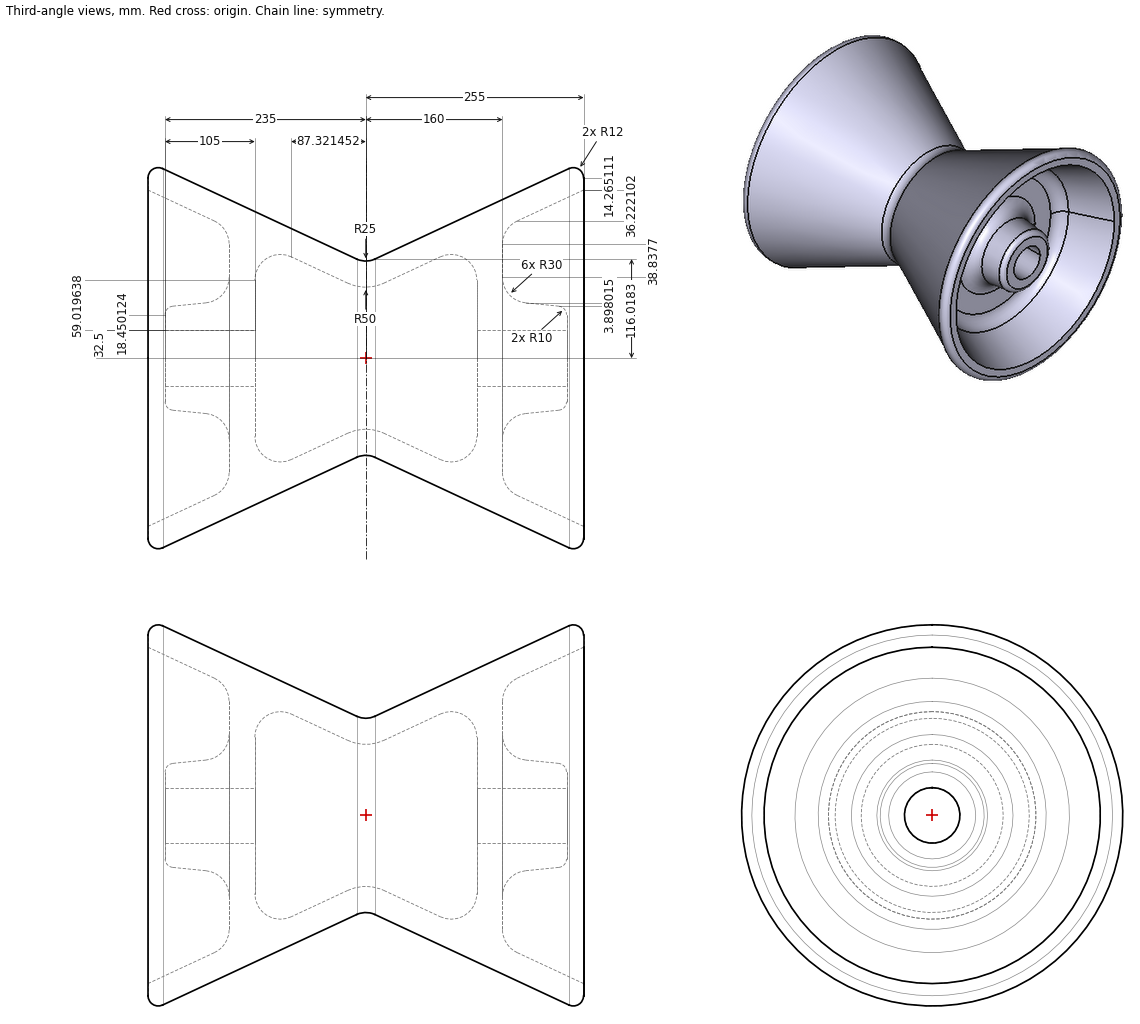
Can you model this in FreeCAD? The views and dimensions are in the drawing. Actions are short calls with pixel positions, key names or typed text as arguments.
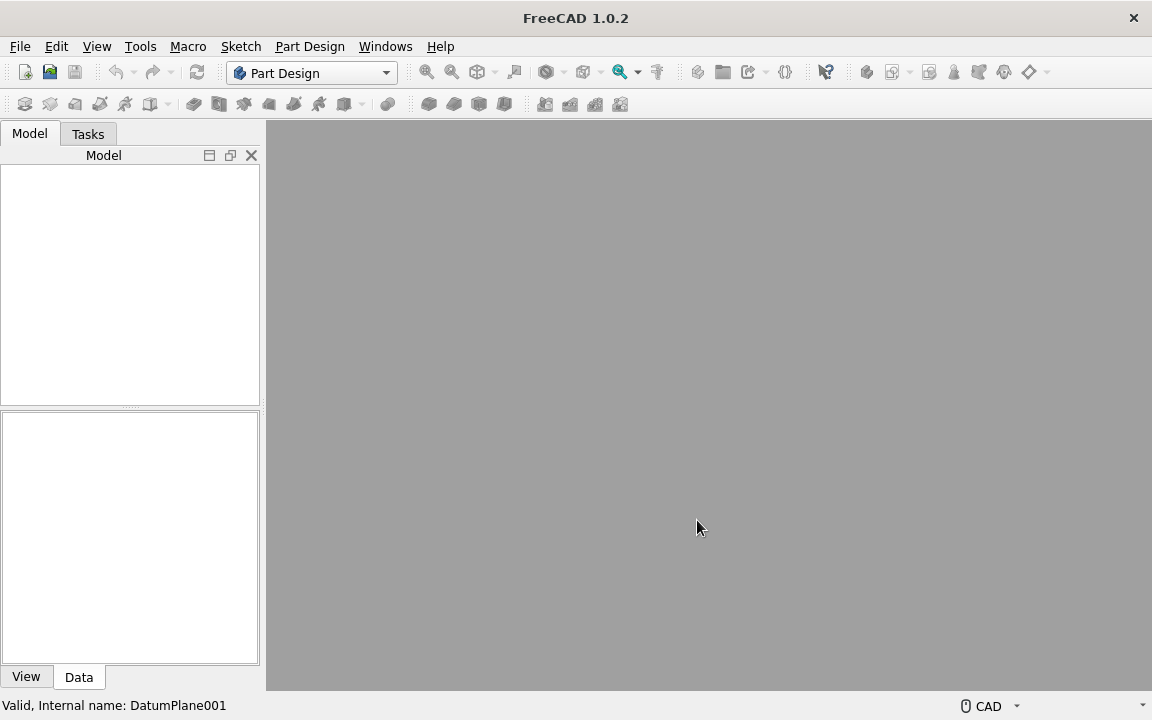
click(25, 72)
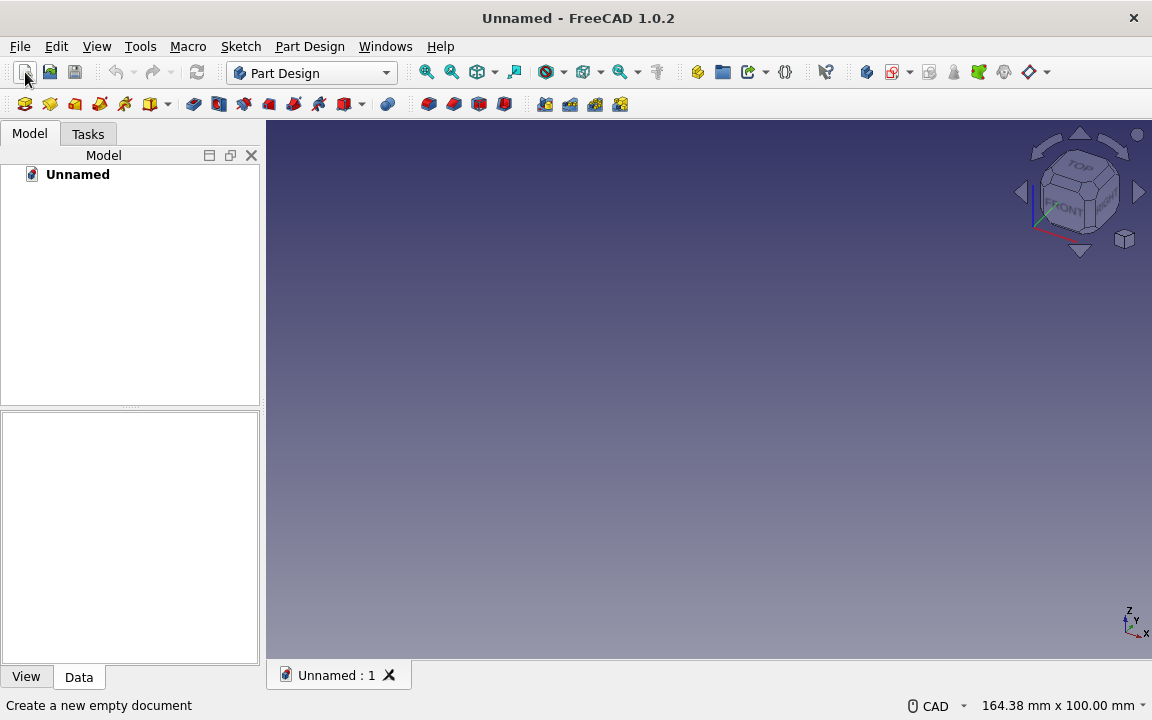
click(892, 72)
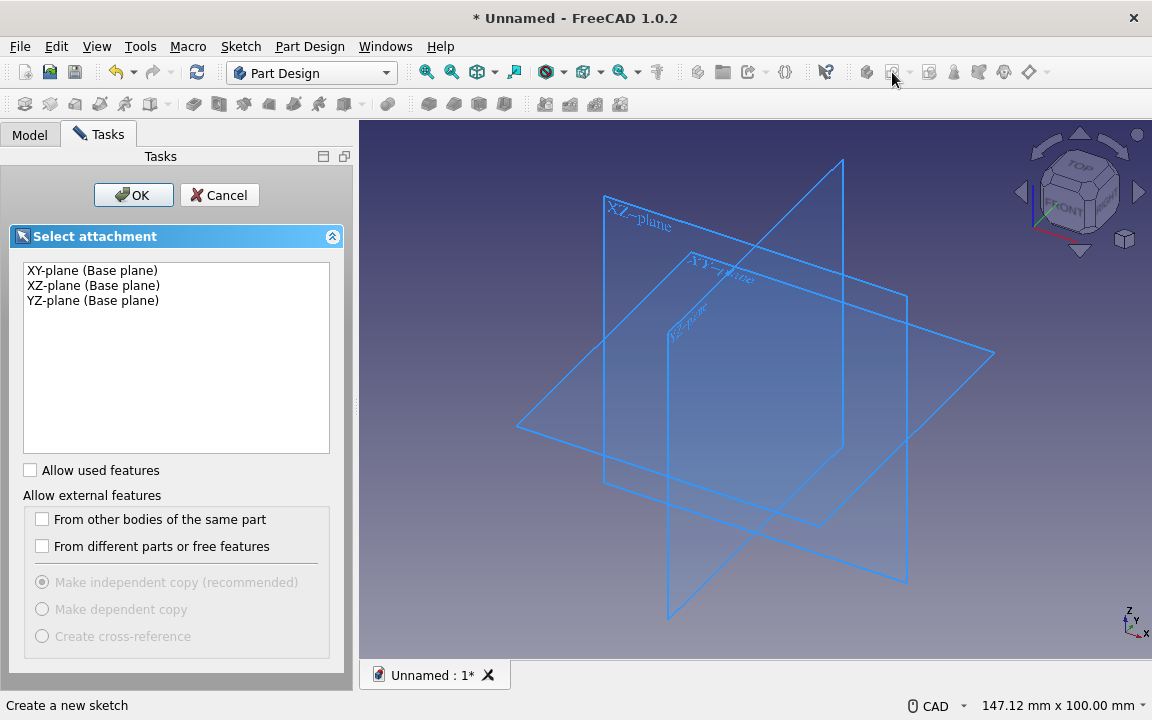
click(84, 270)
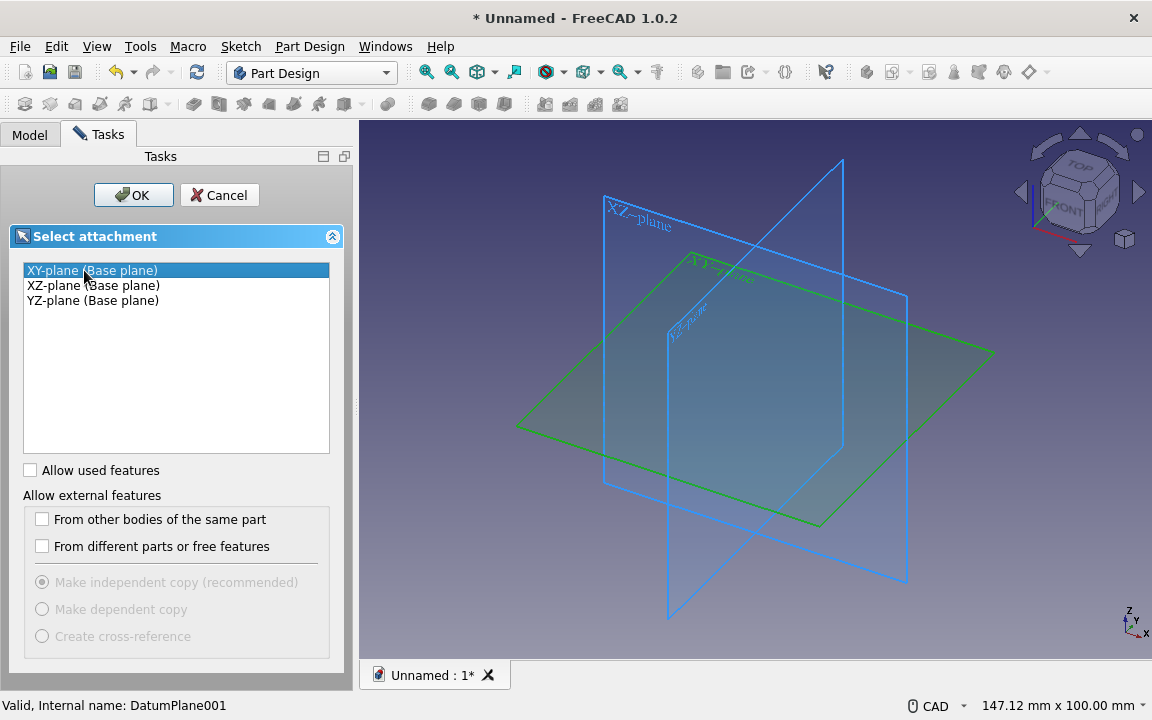
click(134, 195)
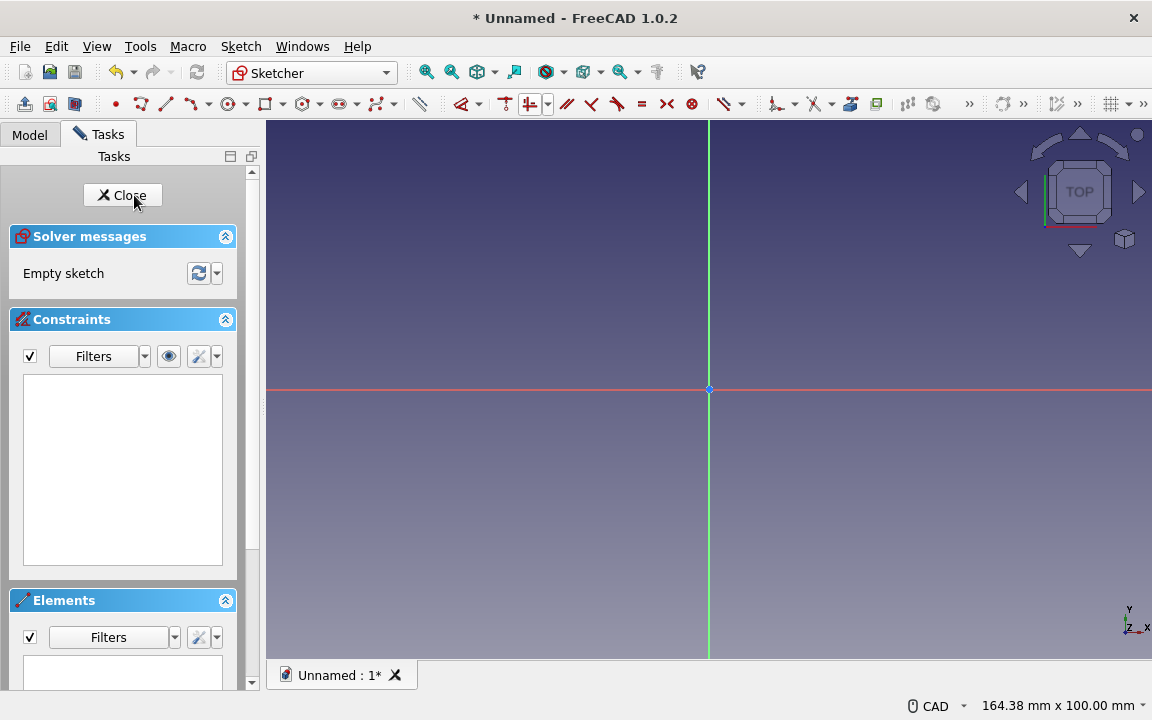
scroll(627, 508, down, 9)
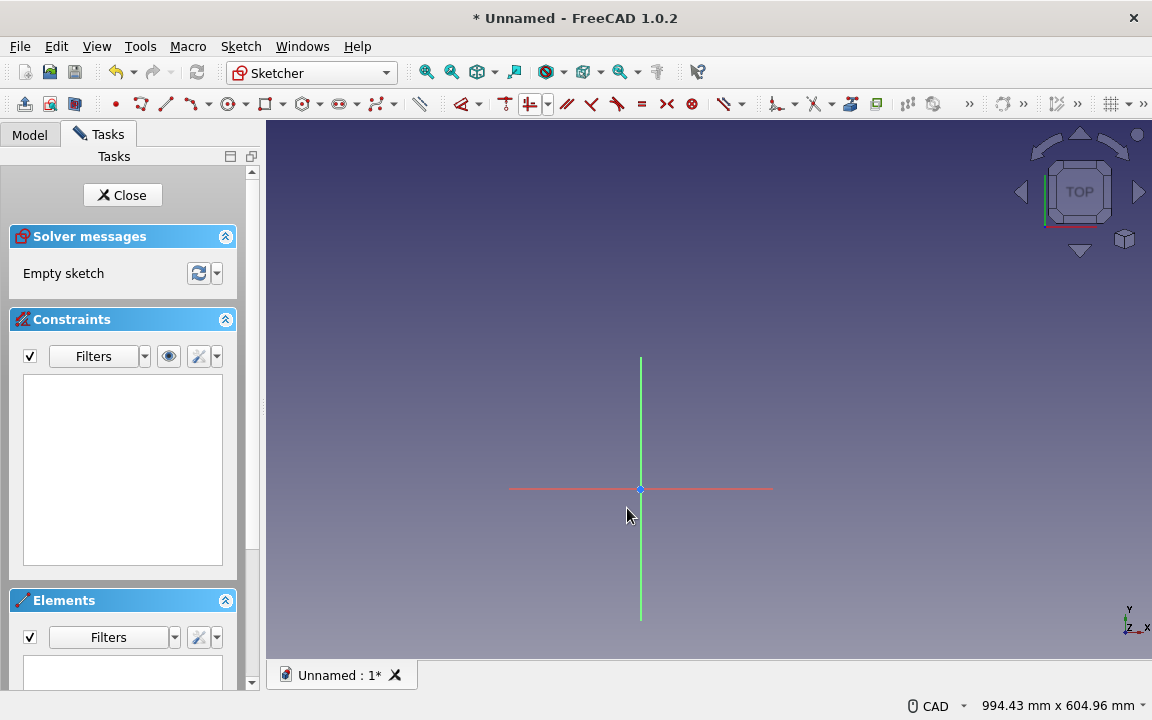
click(166, 104)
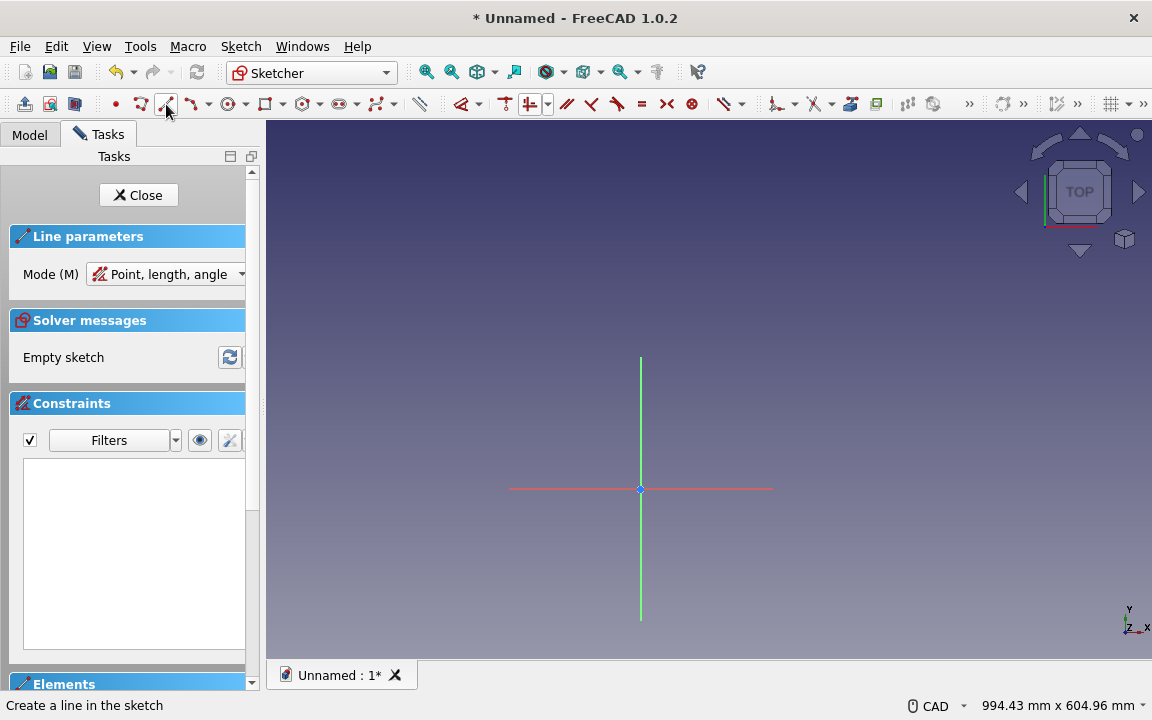
click(842, 435)
click(808, 431)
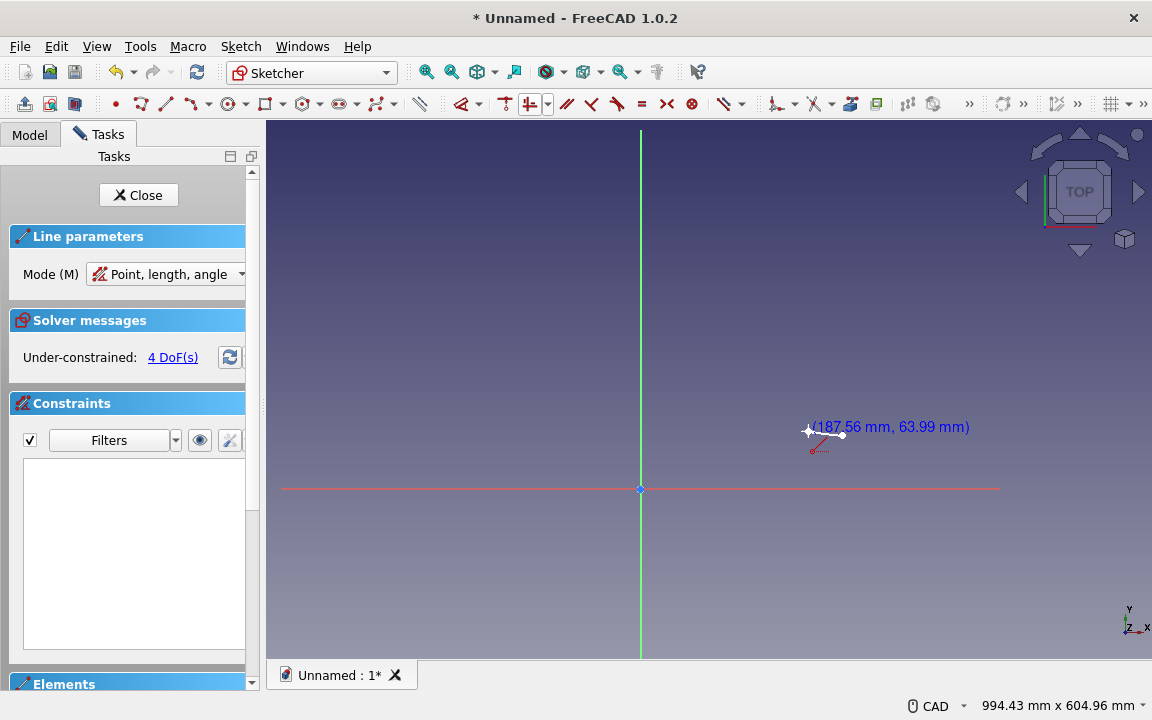
click(783, 405)
click(783, 370)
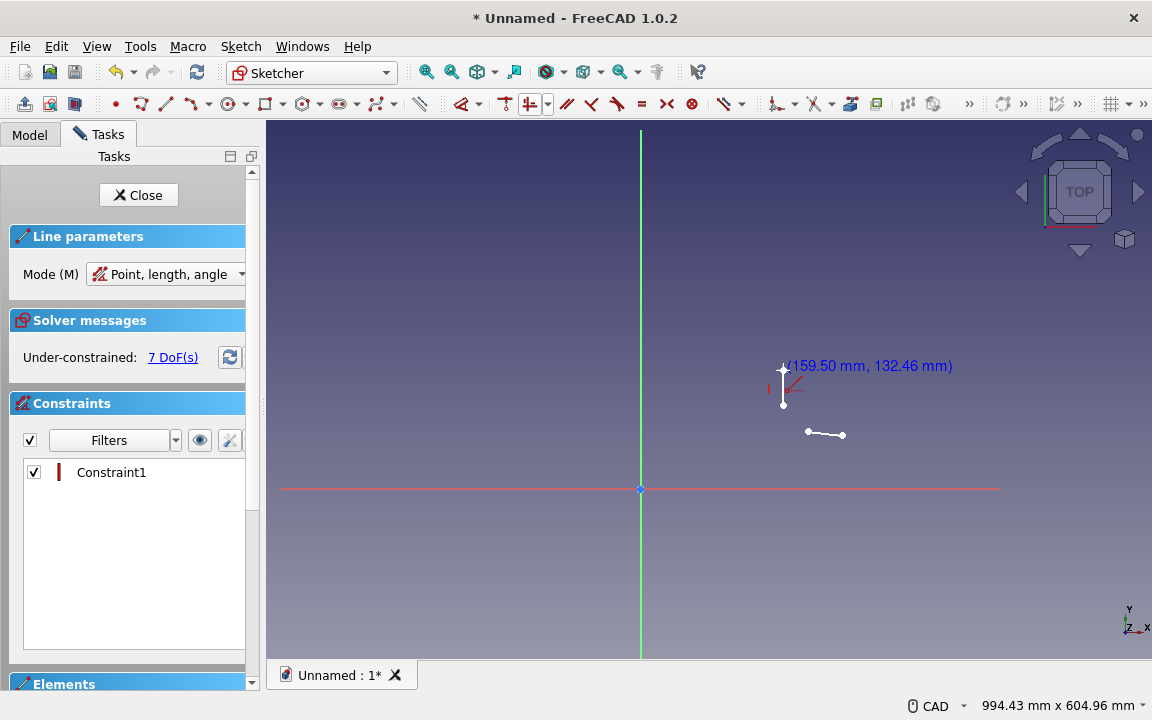
click(141, 104)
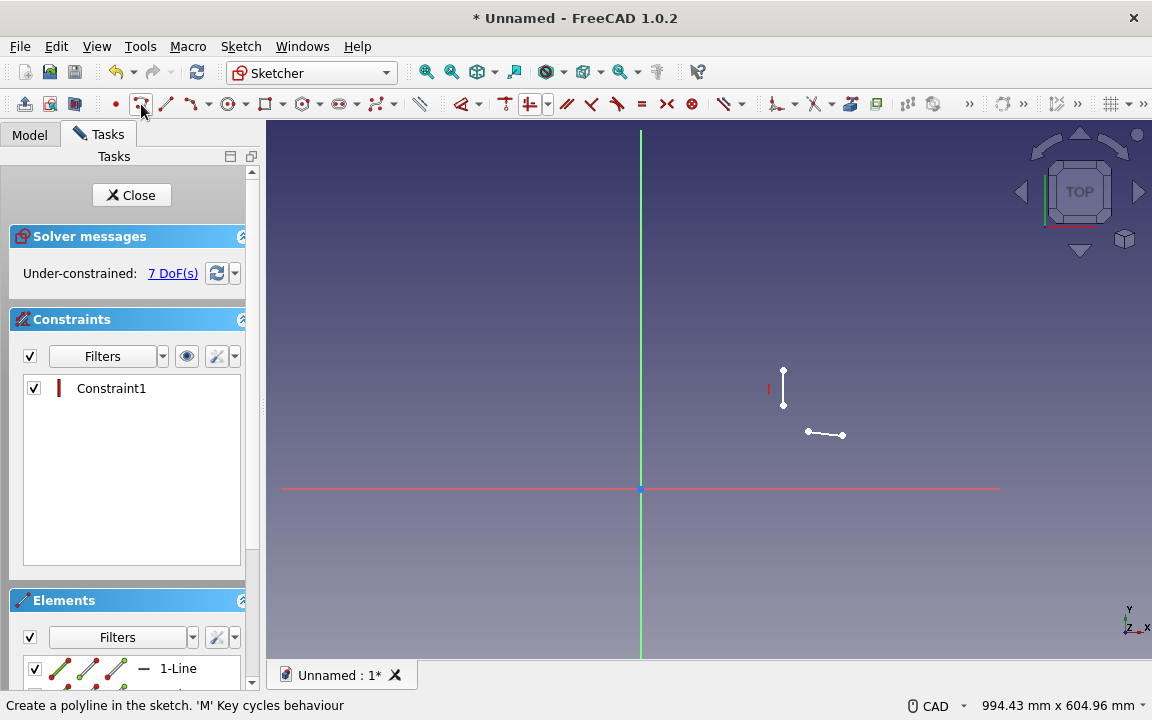
click(799, 346)
click(868, 314)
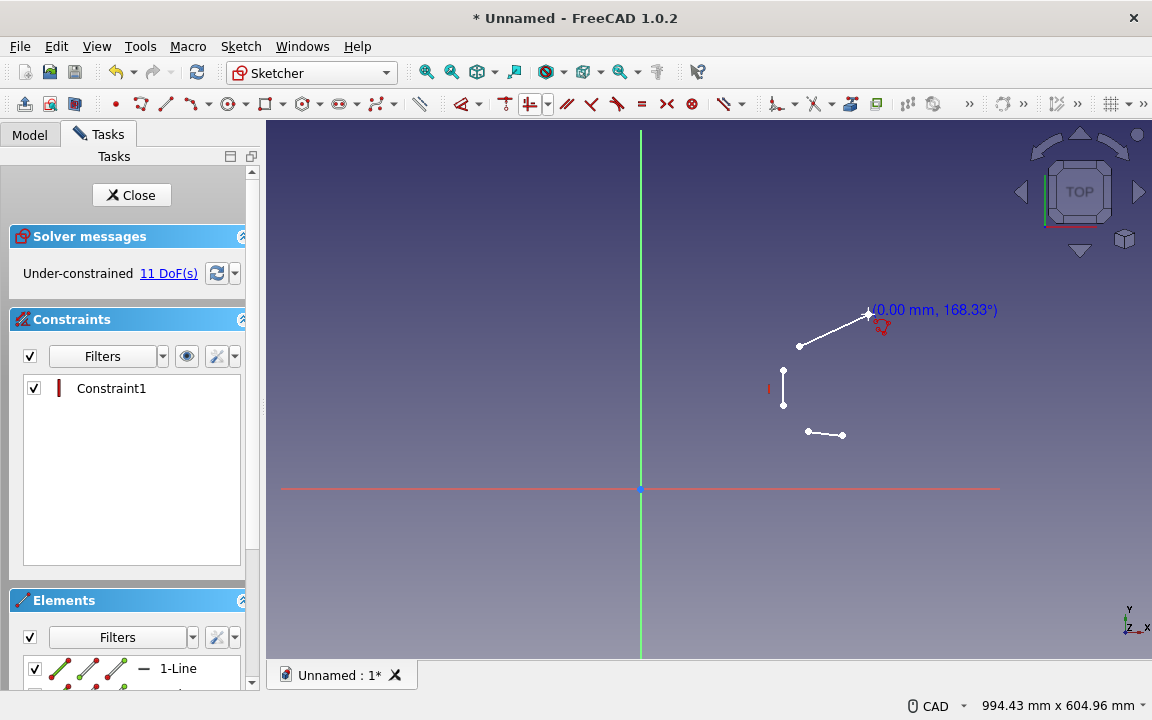
scroll(868, 301, up, 2)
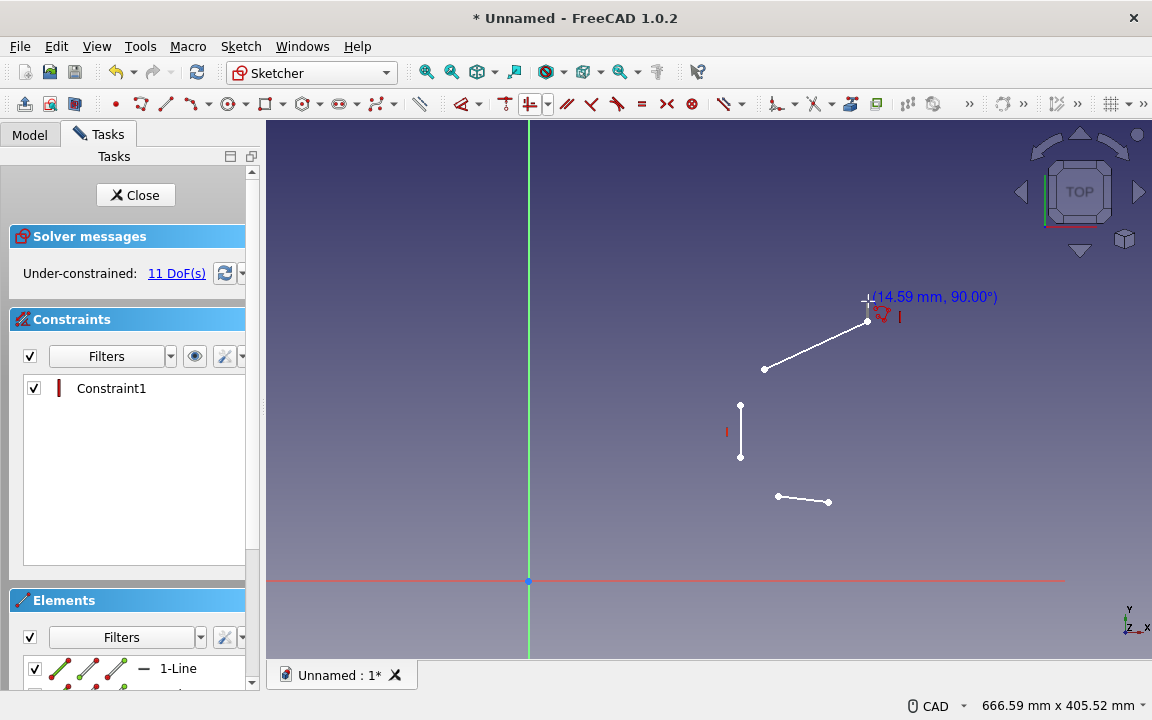
click(868, 301)
right_click(868, 301)